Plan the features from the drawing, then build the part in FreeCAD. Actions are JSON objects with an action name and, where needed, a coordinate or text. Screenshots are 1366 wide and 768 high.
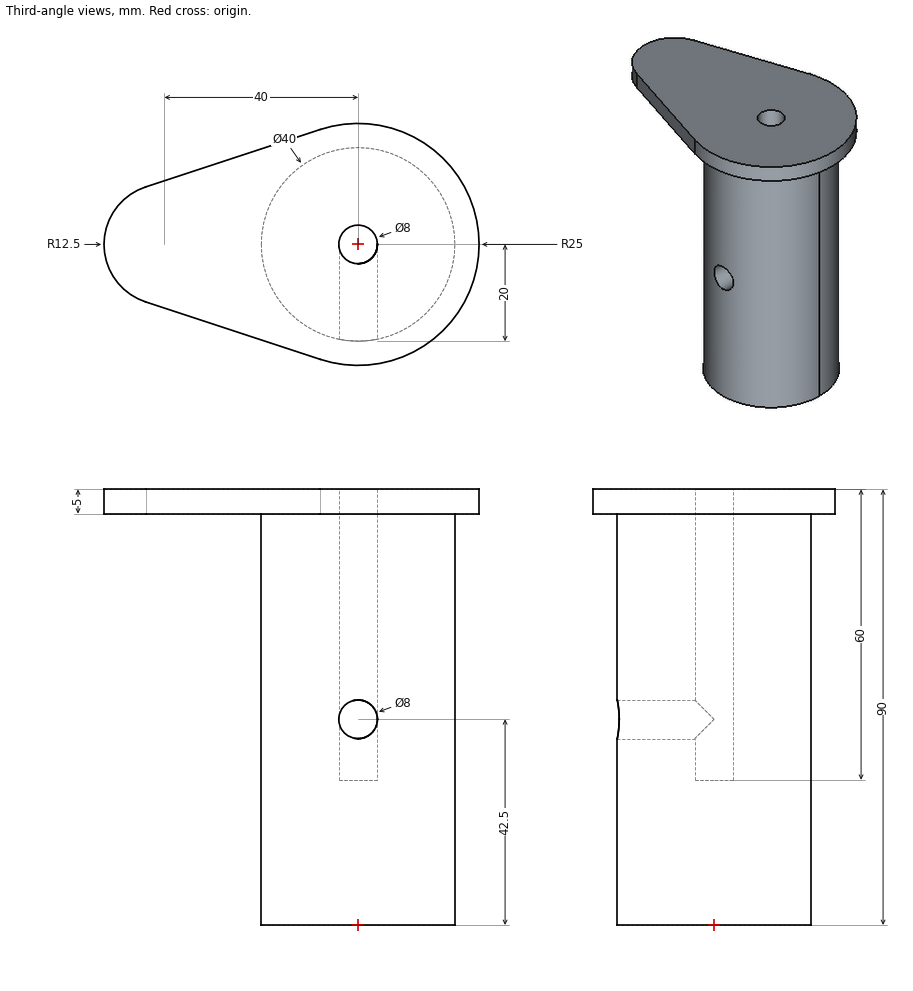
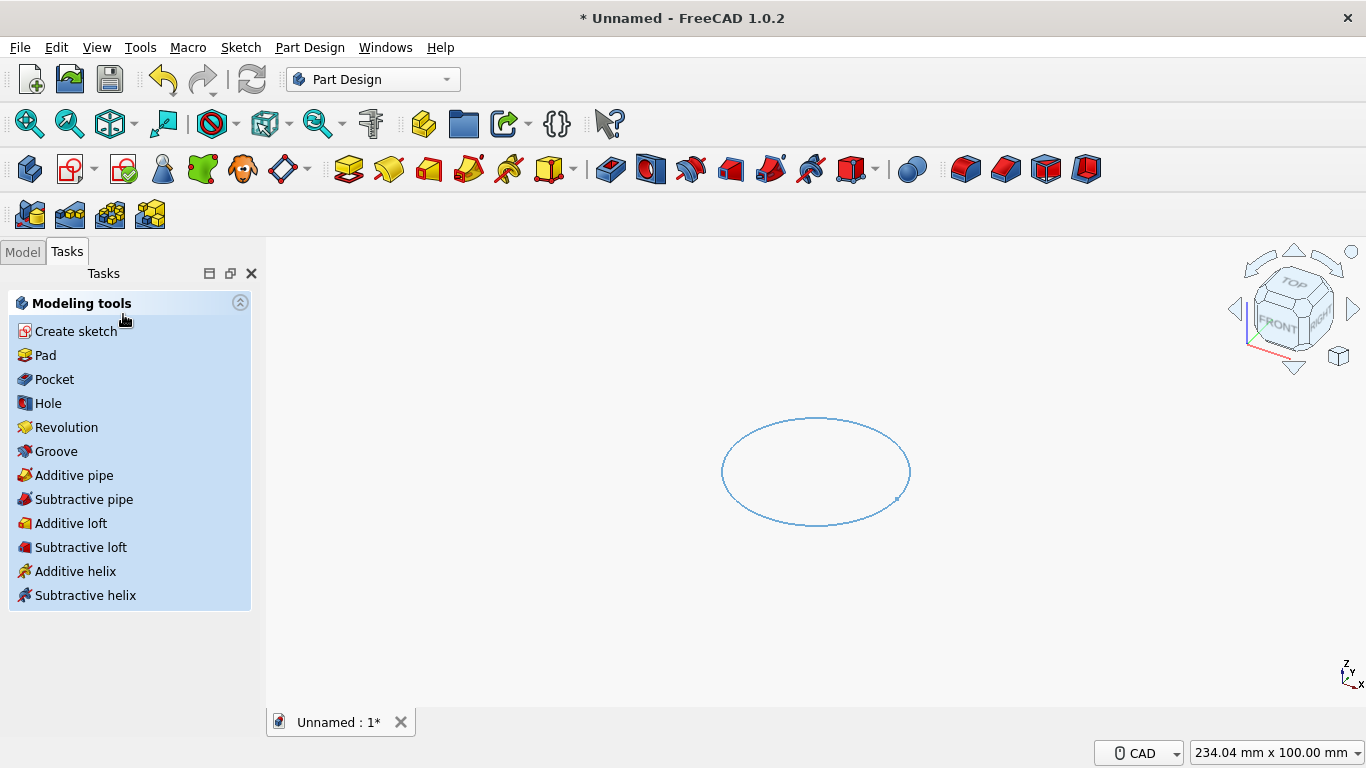
{"action": "left_click", "coordinate": [350, 170]}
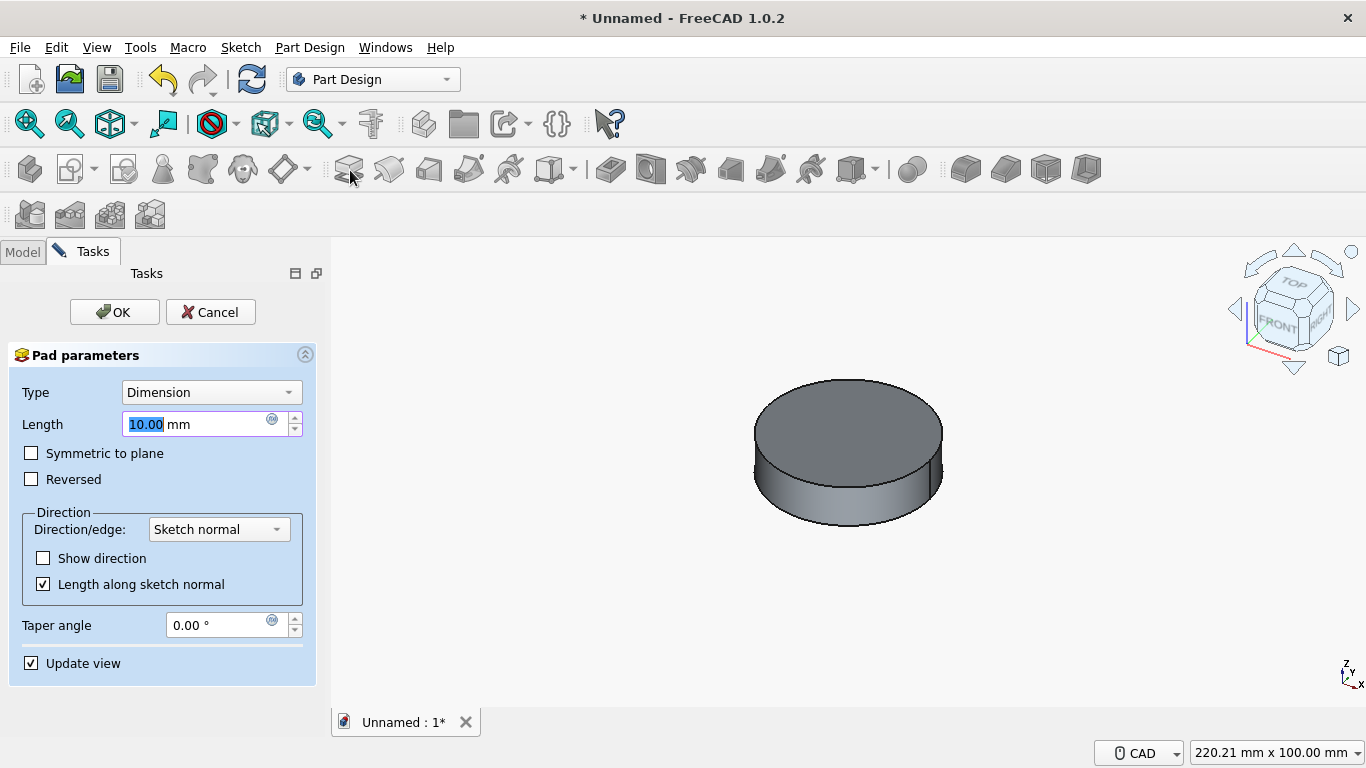
{"action": "type", "text": "90"}
{"action": "key", "text": "Tab"}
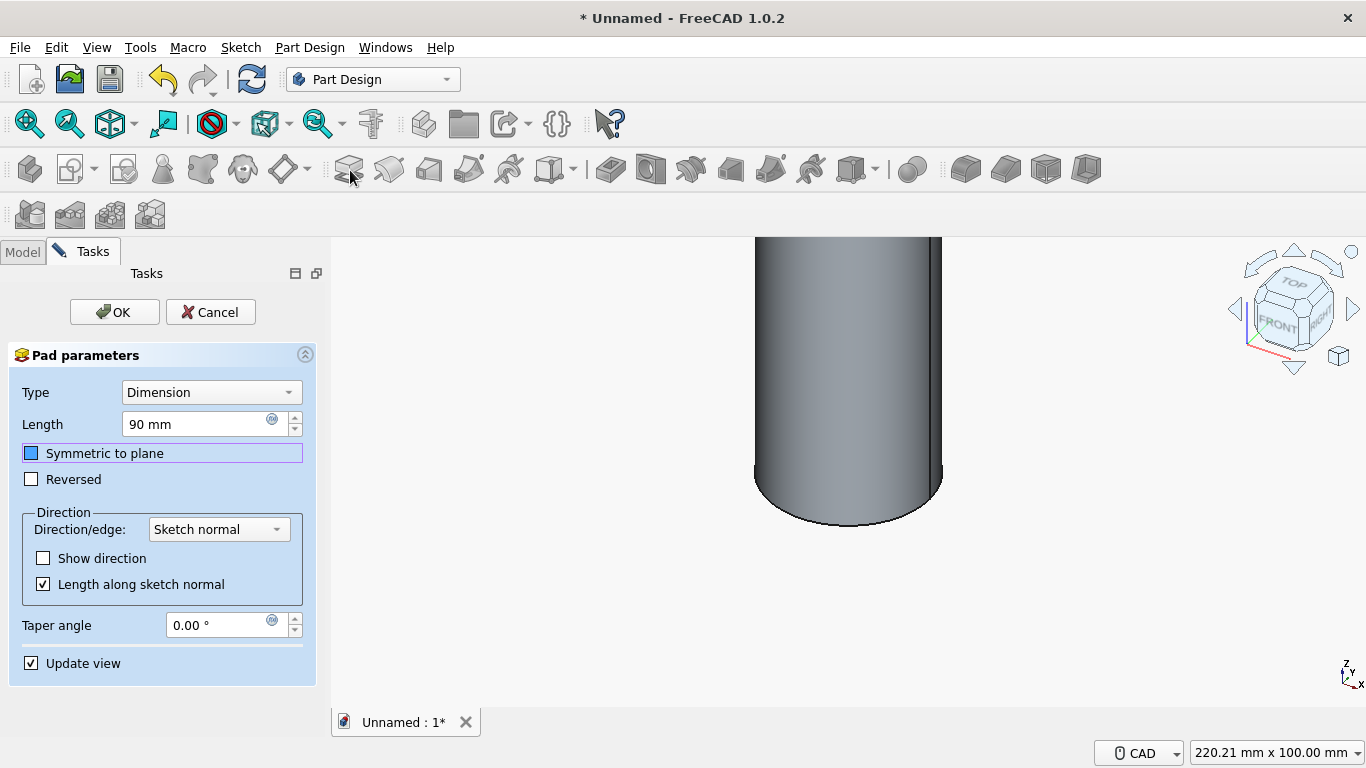
{"action": "left_click", "coordinate": [115, 312]}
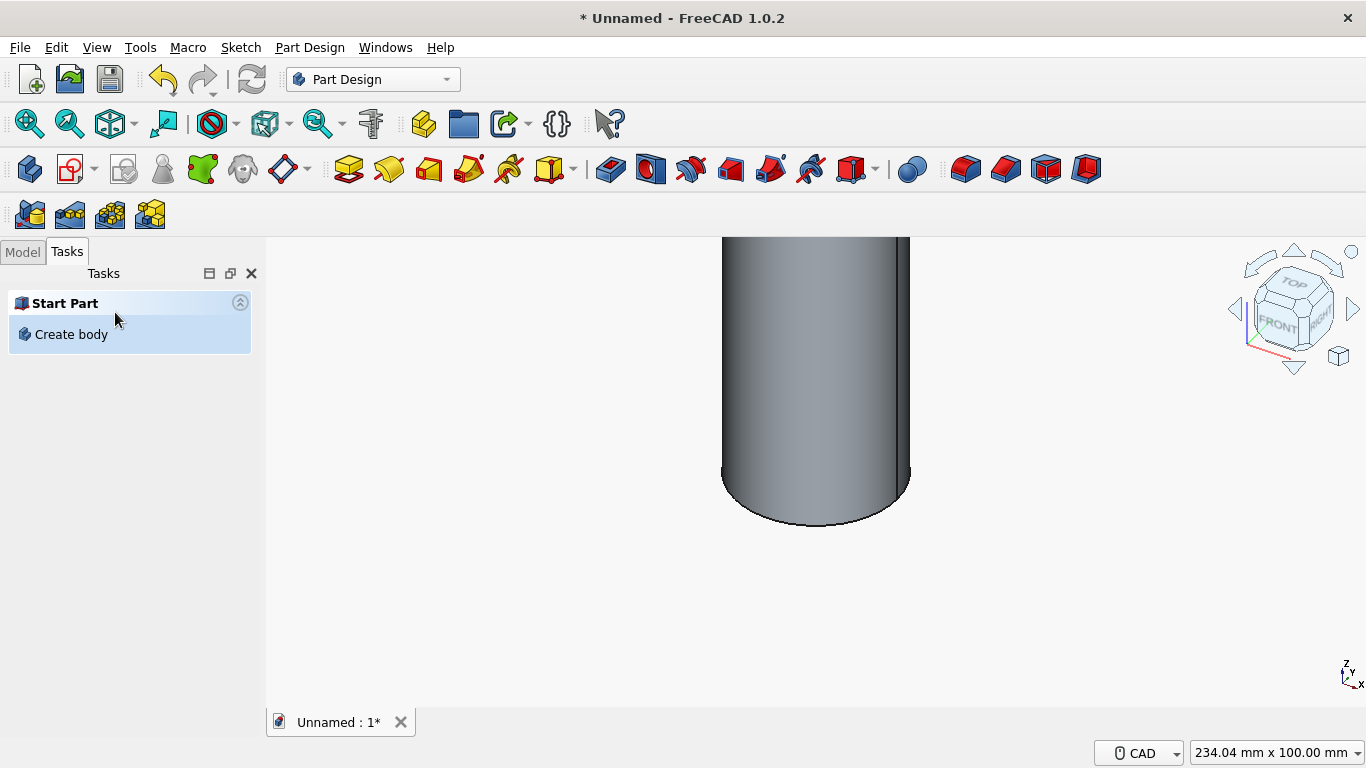
{"action": "key", "text": "v f"}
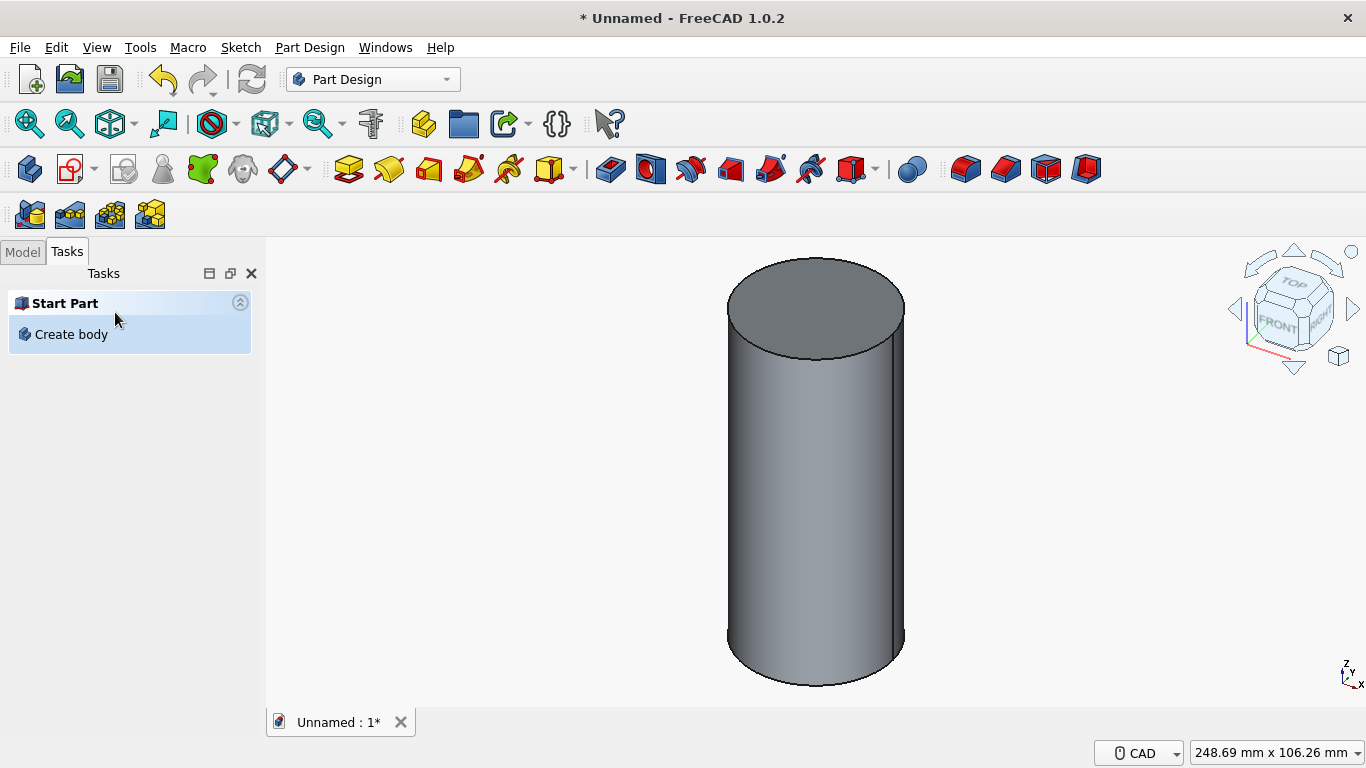
{"action": "left_click", "coordinate": [816, 308]}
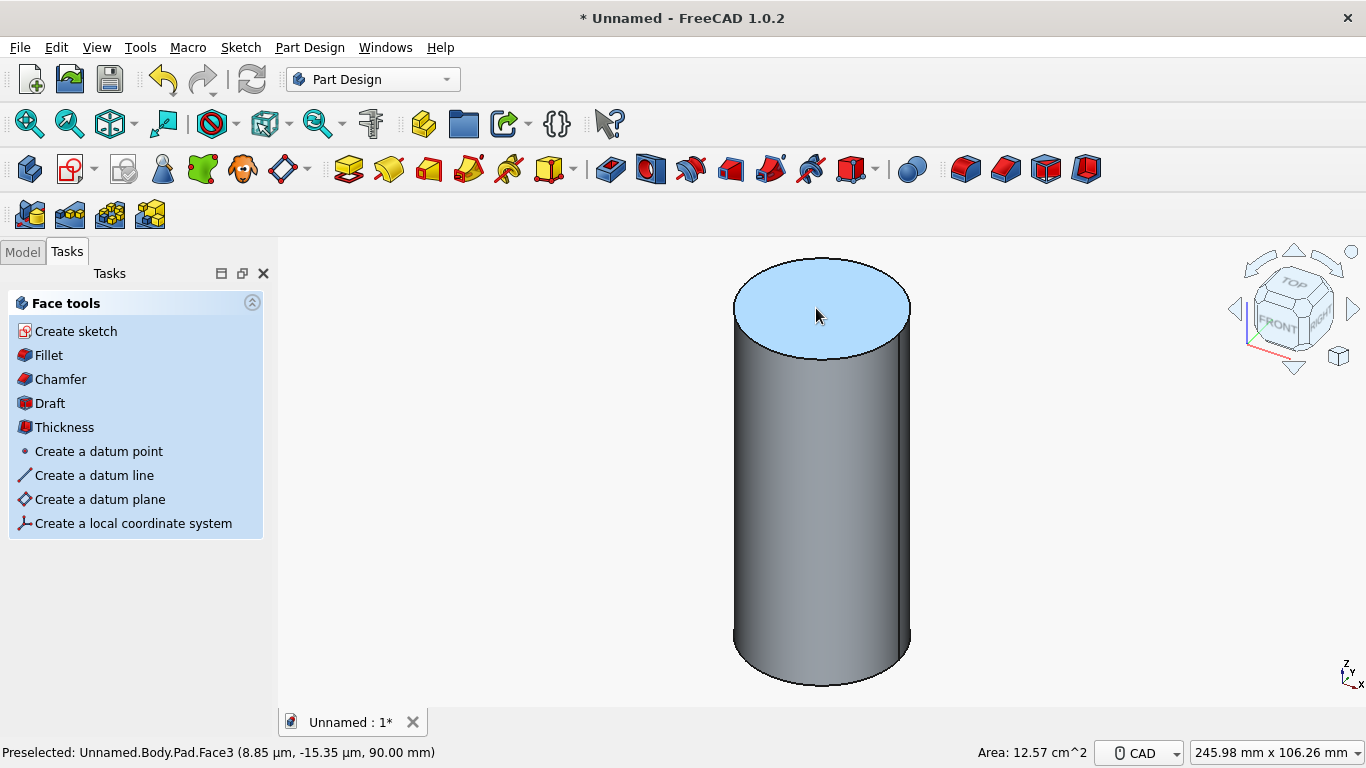
{"action": "left_click", "coordinate": [70, 170]}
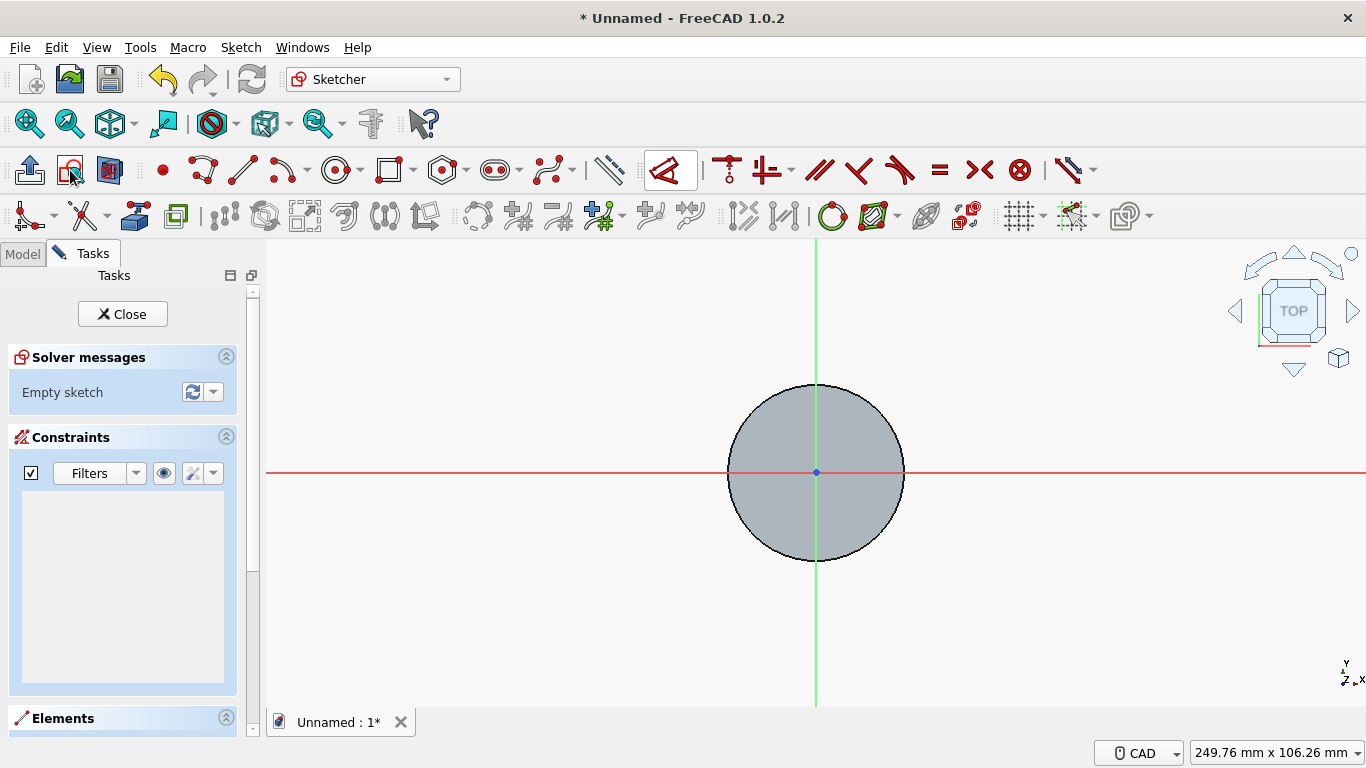
{"action": "scroll", "coordinate": [772, 473], "scroll_direction": "up", "scroll_amount": 2}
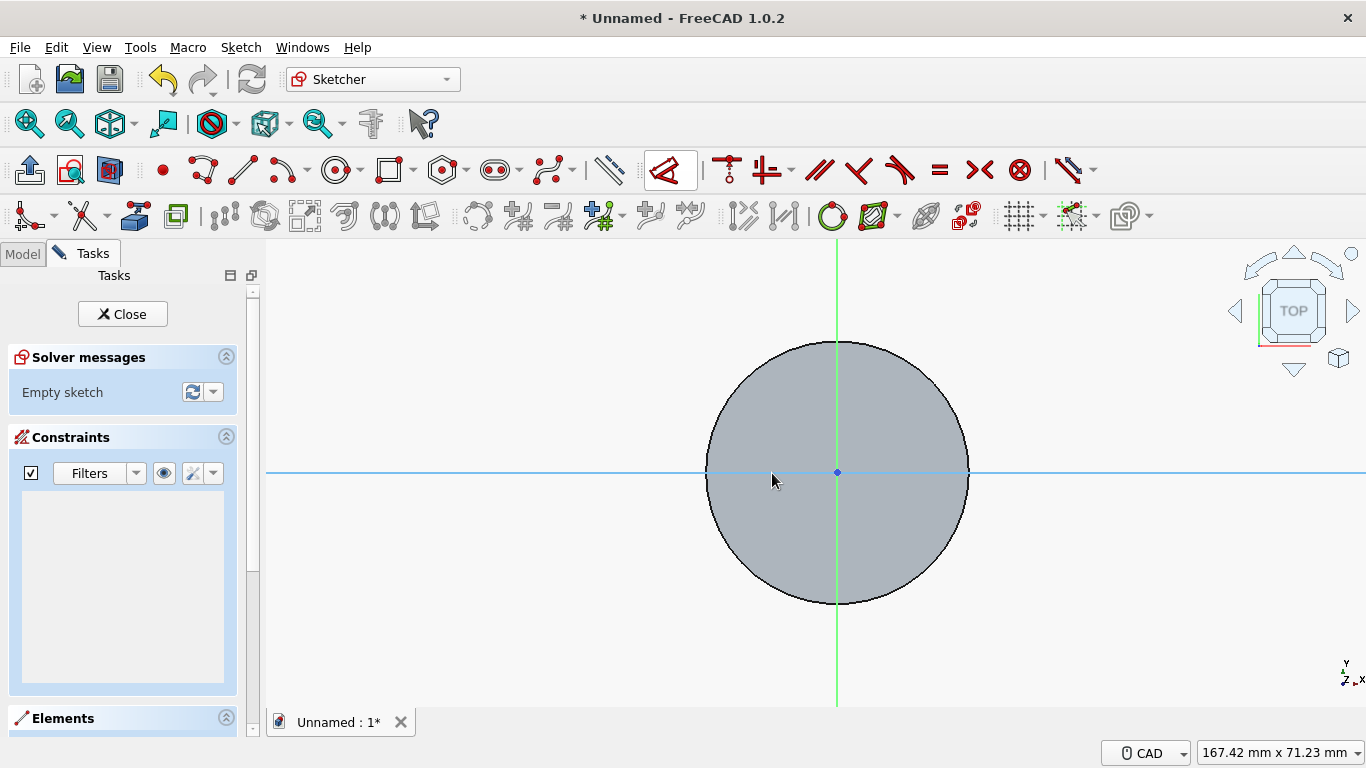
{"action": "key", "text": "g l"}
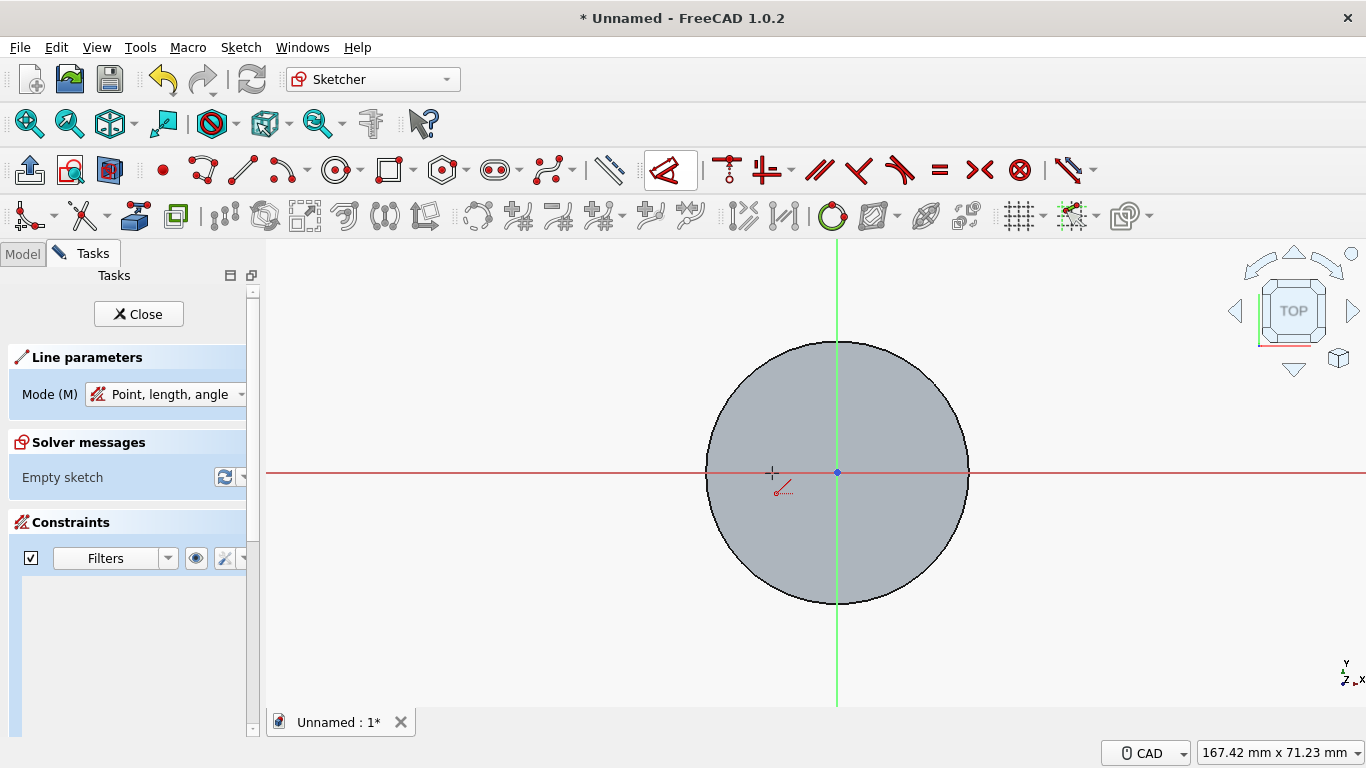
{"action": "left_click", "coordinate": [786, 317]}
{"action": "left_click", "coordinate": [549, 395]}